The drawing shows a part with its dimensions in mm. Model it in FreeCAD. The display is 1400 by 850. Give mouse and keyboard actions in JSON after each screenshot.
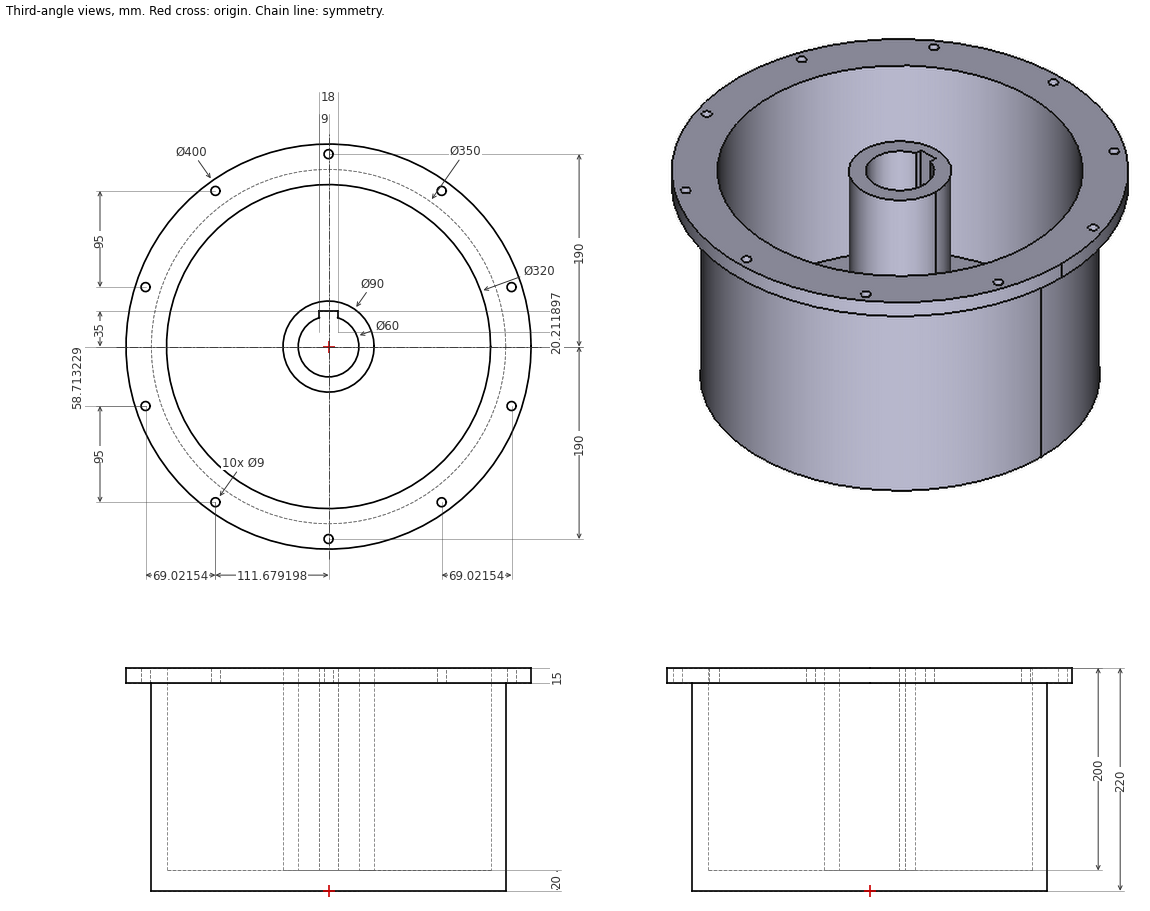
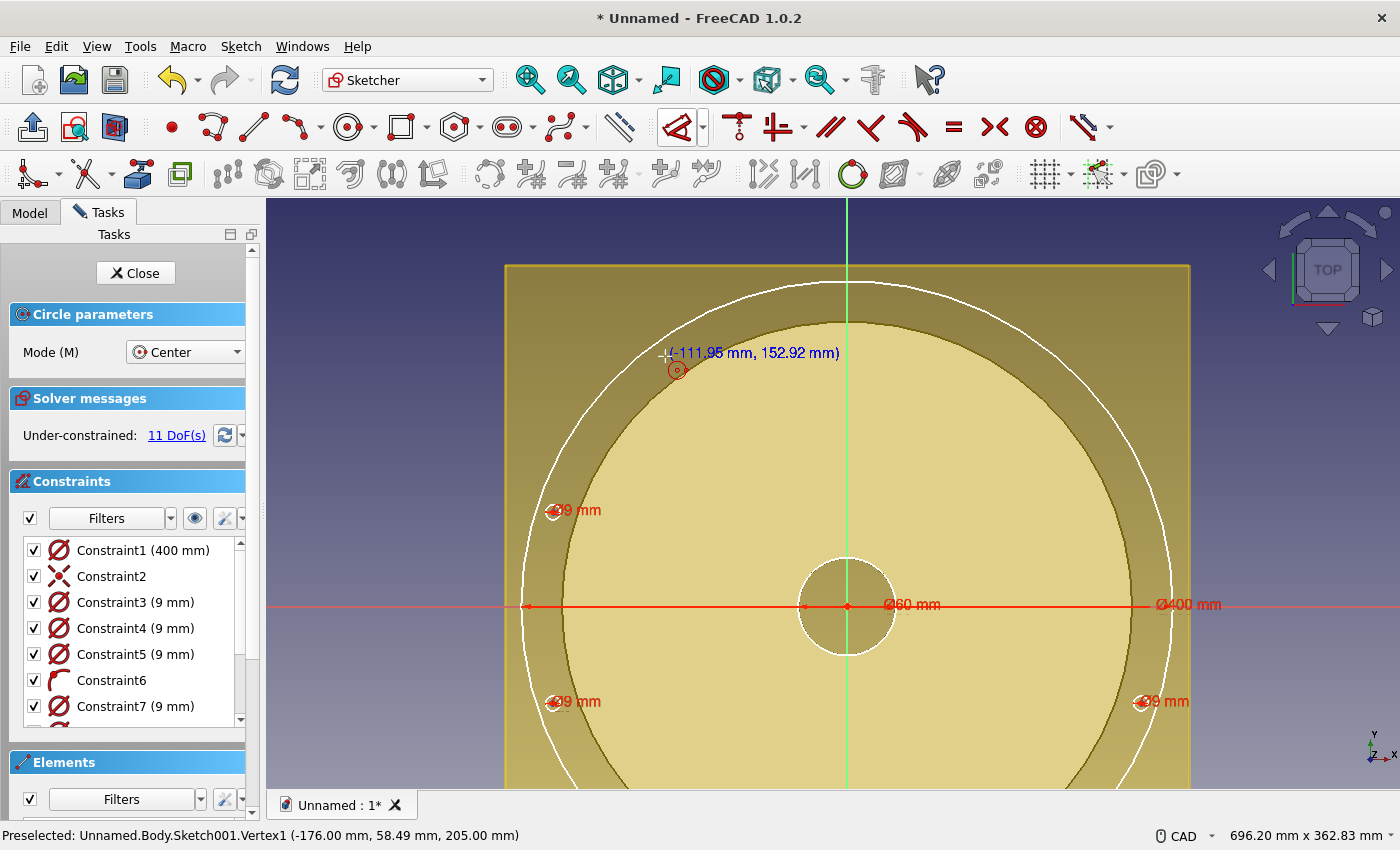
{"action": "left_click", "coordinate": [665, 356]}
{"action": "mouse_move", "coordinate": [670, 351]}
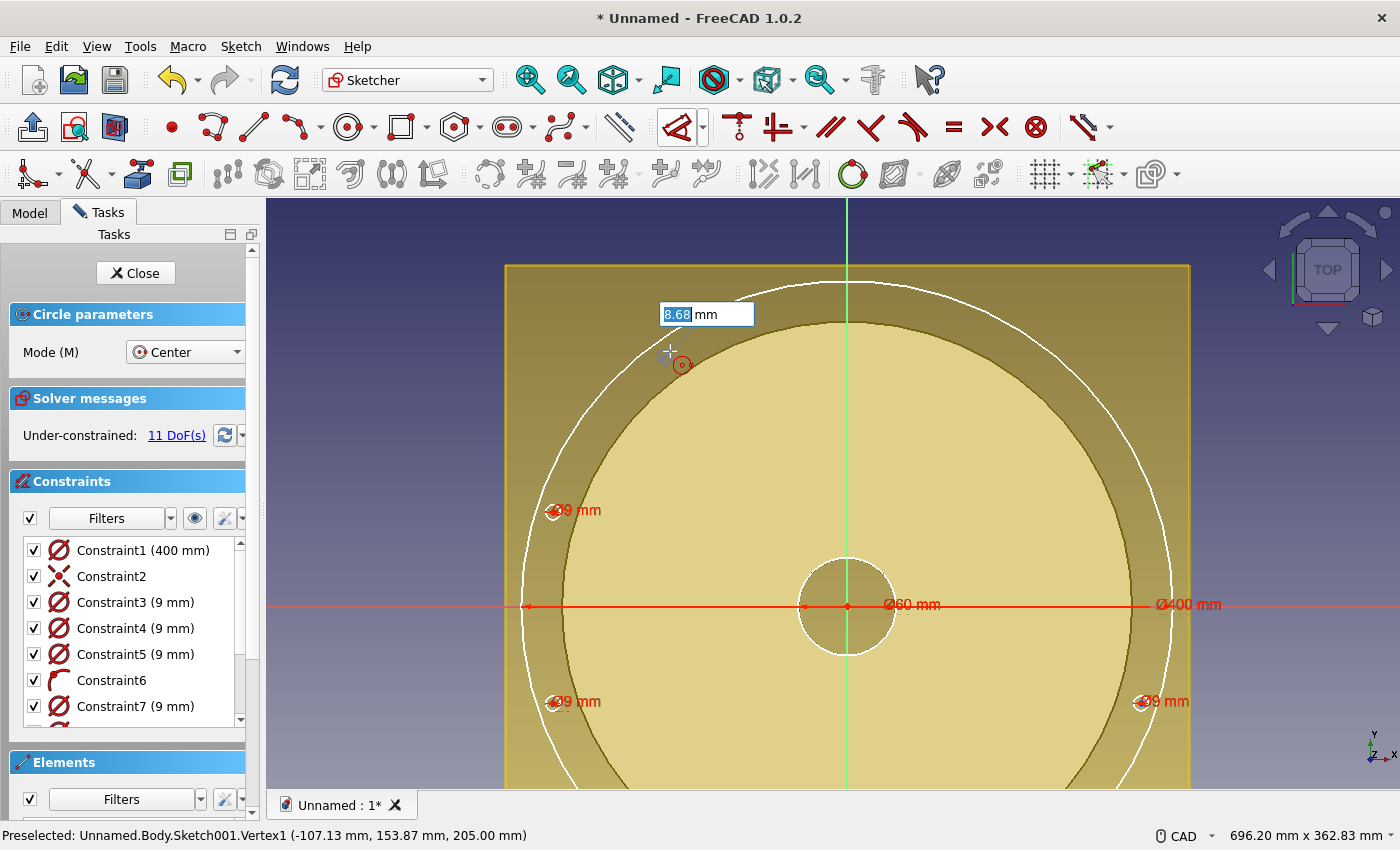
{"action": "type", "text": "9"}
{"action": "key", "text": "Return"}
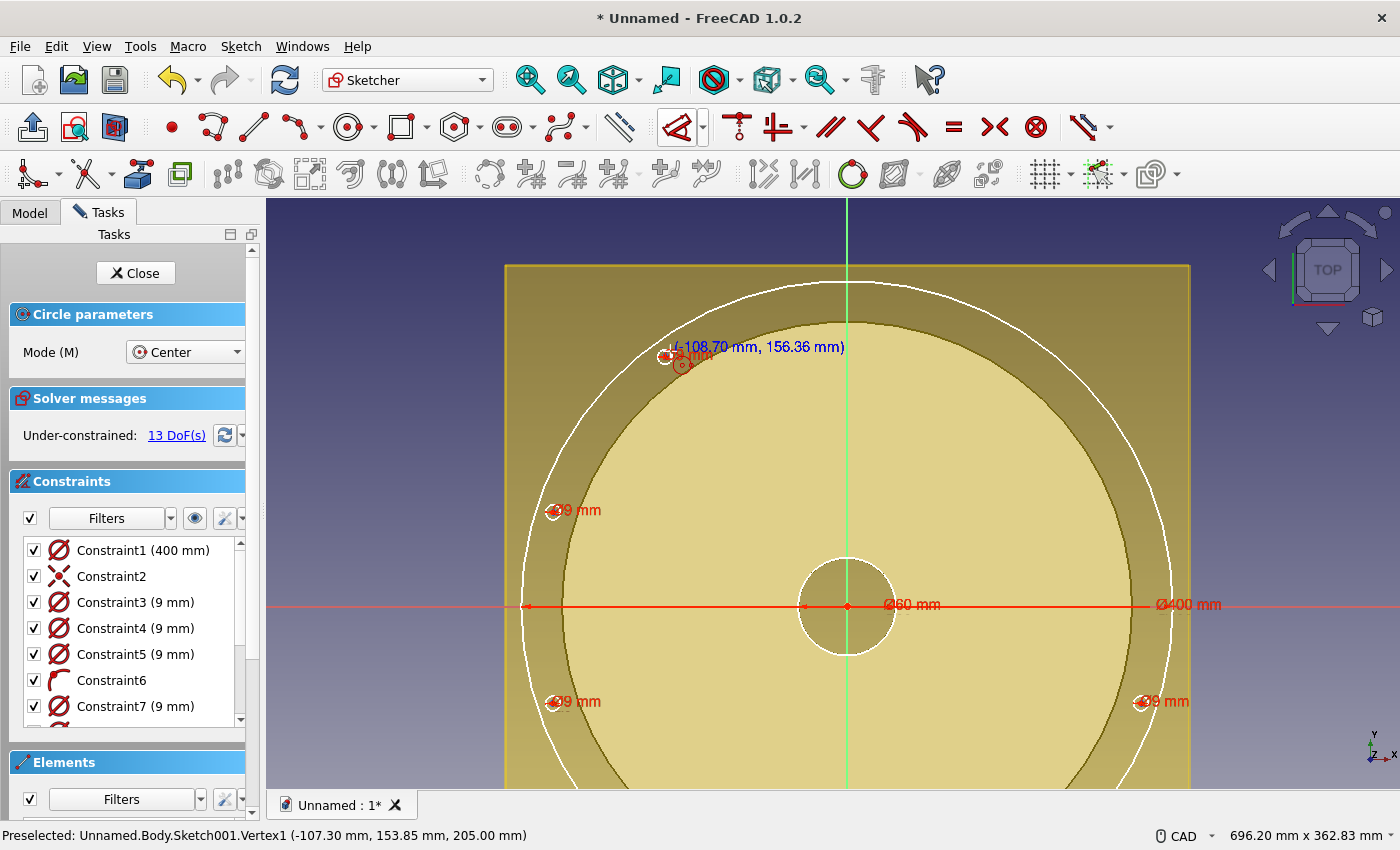
{"action": "scroll", "coordinate": [1141, 511], "scroll_direction": "up", "scroll_amount": 6}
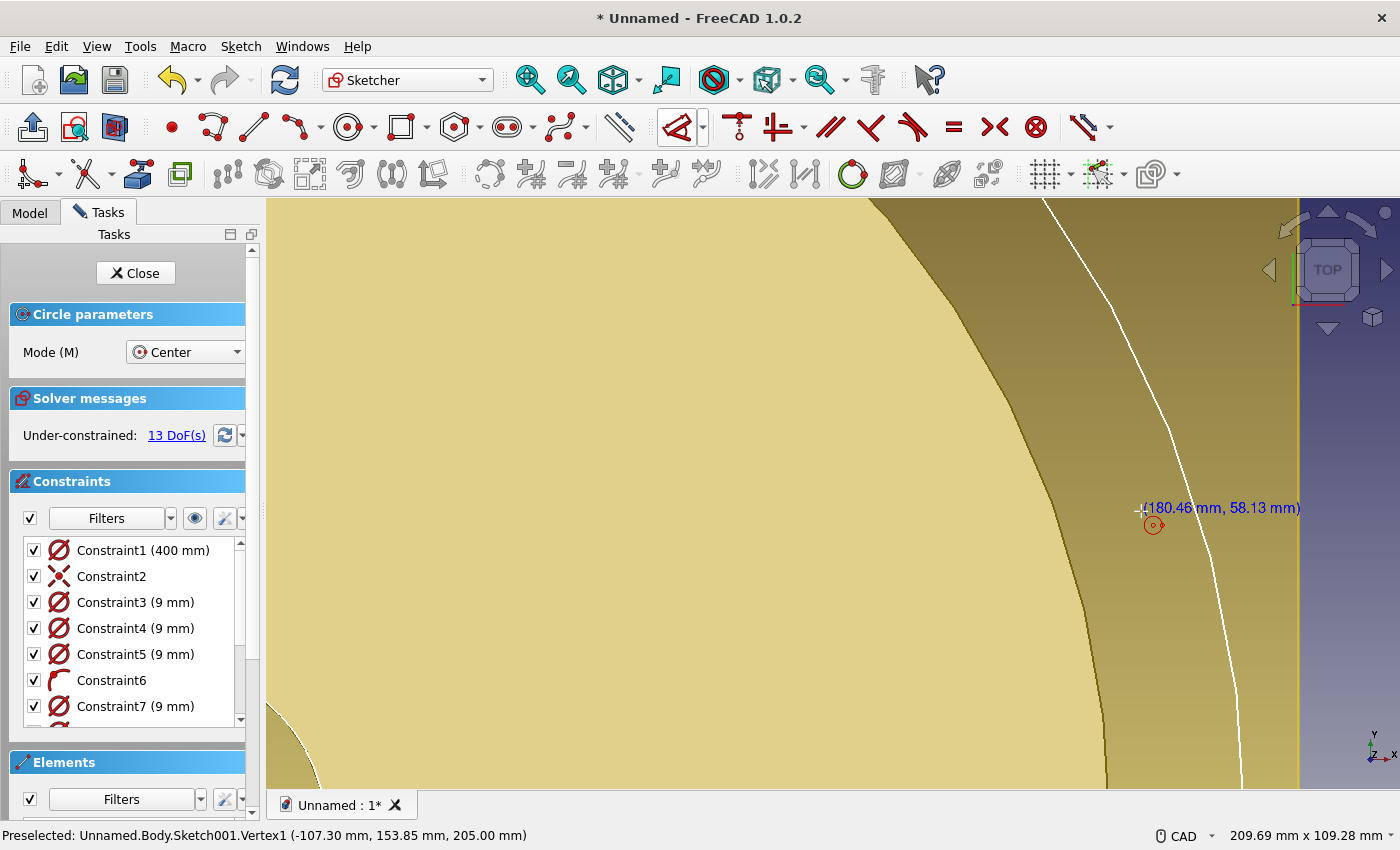
{"action": "scroll", "coordinate": [884, 427], "scroll_direction": "down", "scroll_amount": 9}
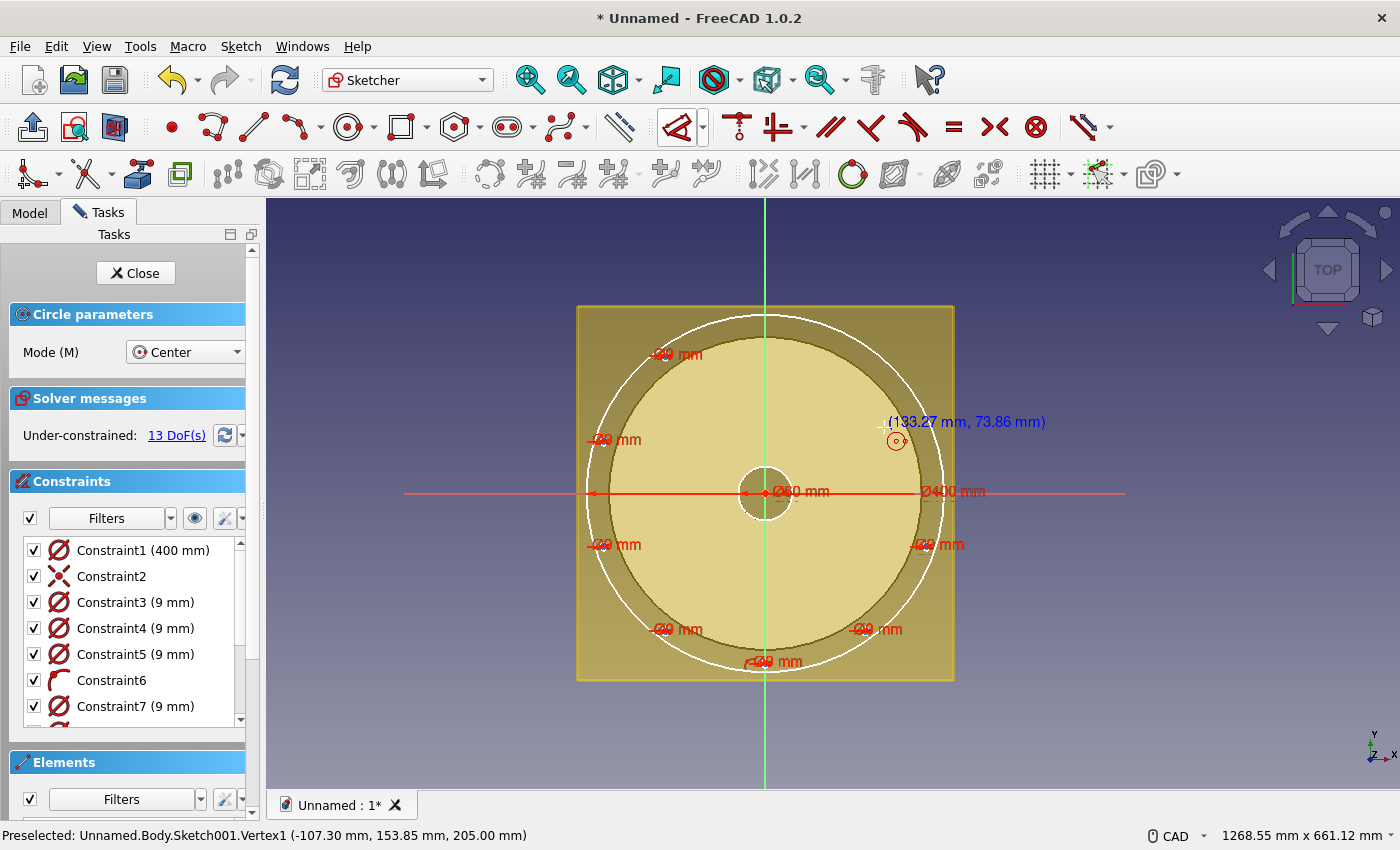
{"action": "scroll", "coordinate": [927, 441], "scroll_direction": "up", "scroll_amount": 3}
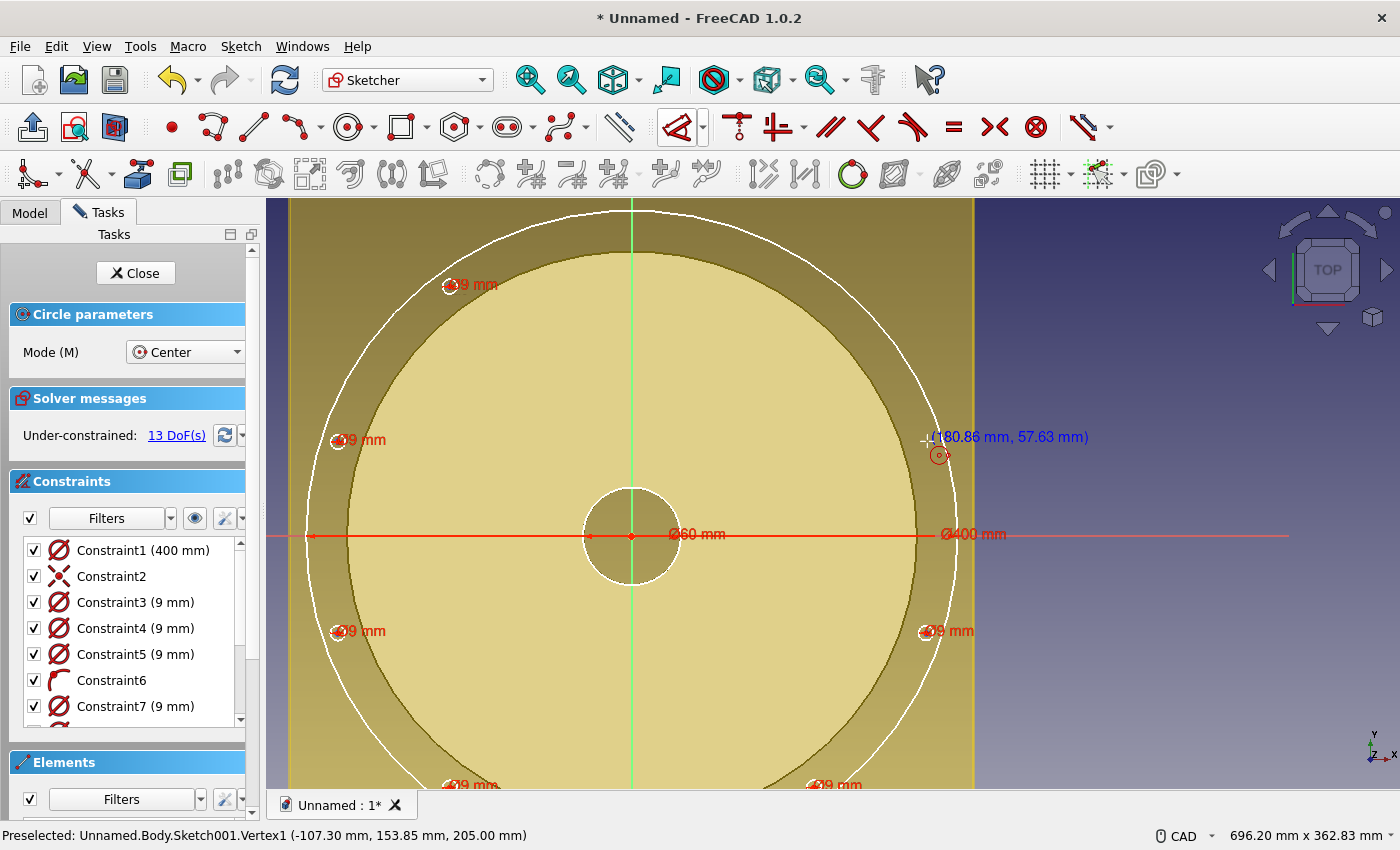
{"action": "left_click", "coordinate": [926, 441]}
{"action": "mouse_move", "coordinate": [921, 436]}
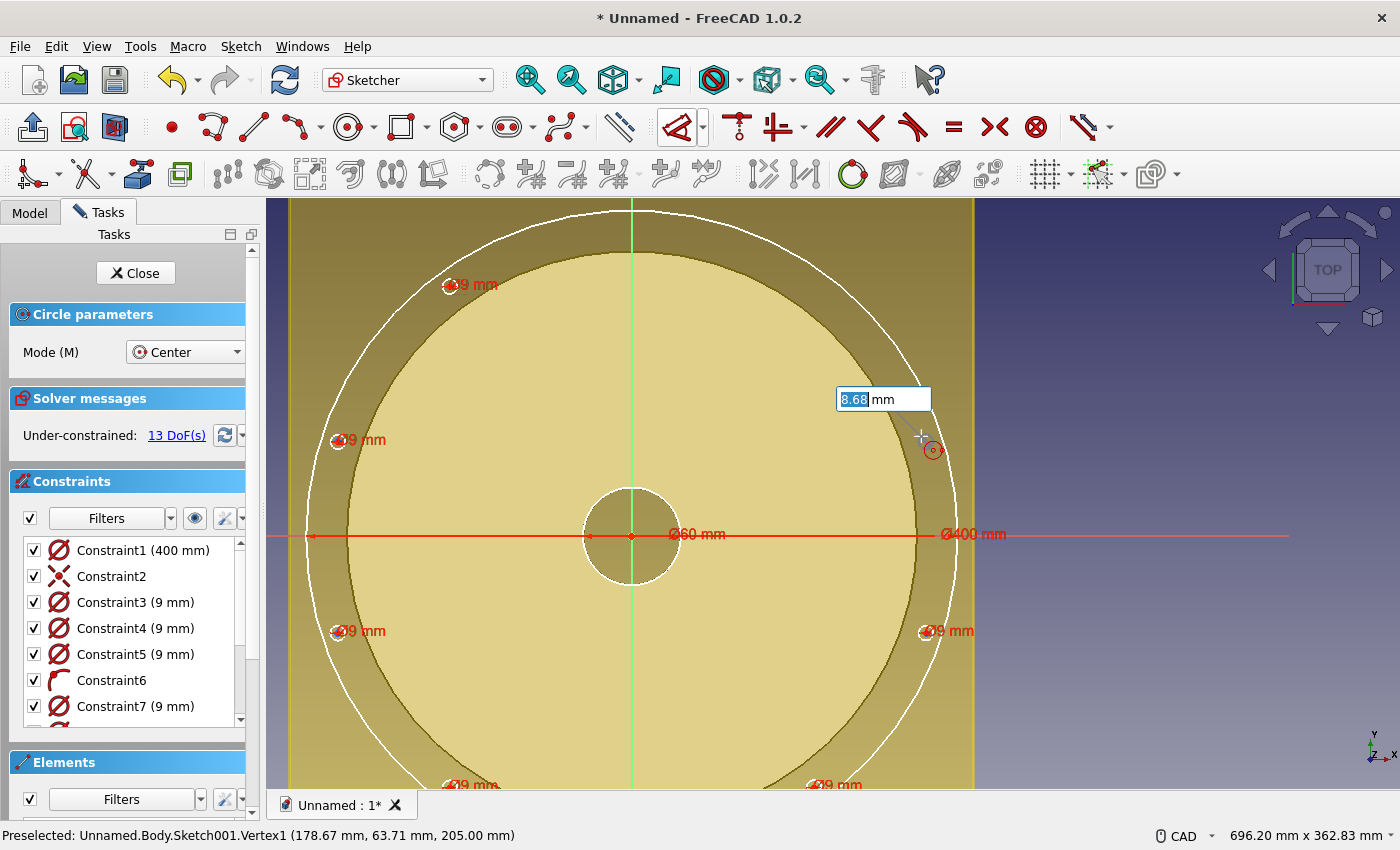
{"action": "type", "text": "9"}
{"action": "key", "text": "Return"}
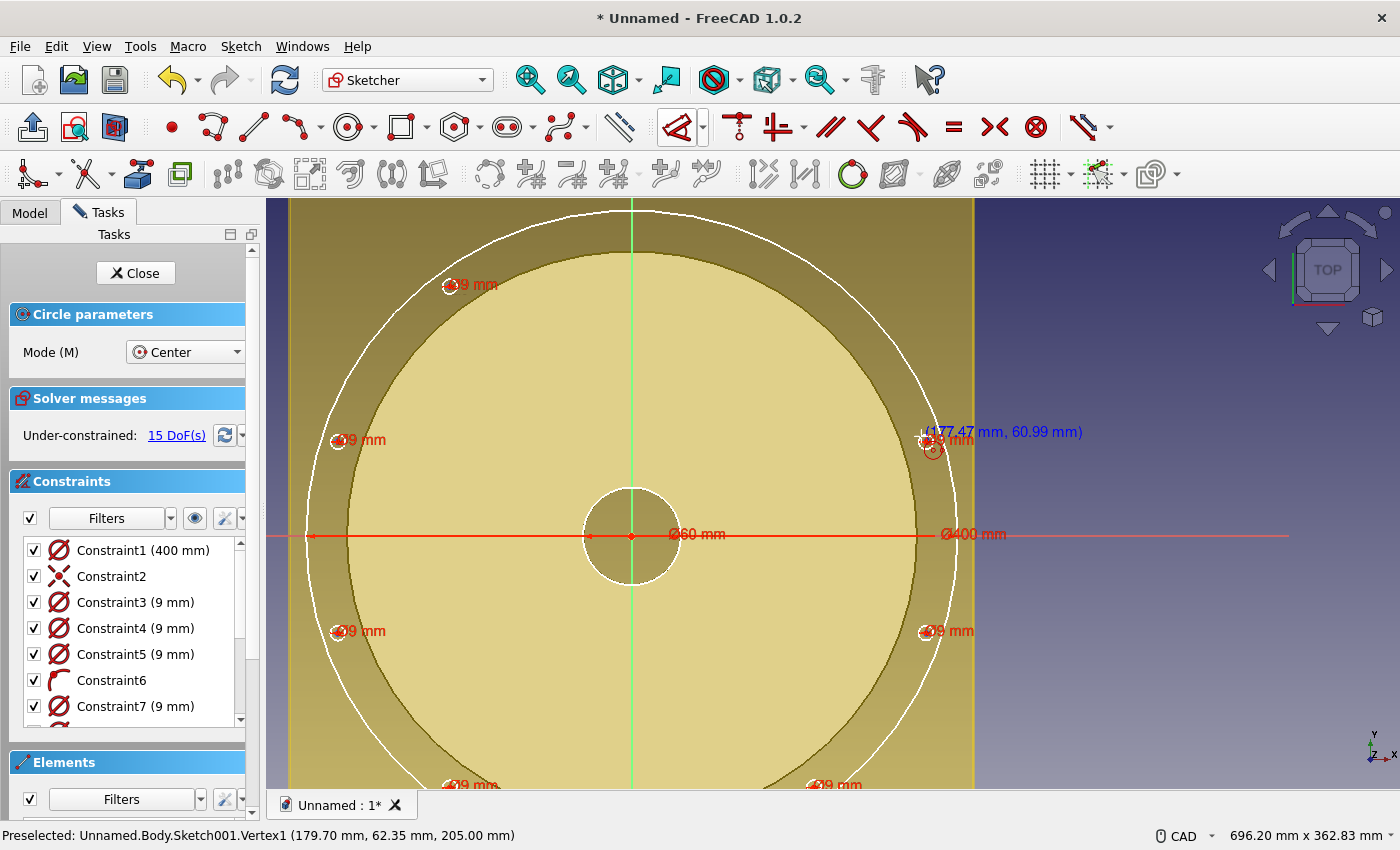
{"action": "scroll", "coordinate": [632, 227], "scroll_direction": "up", "scroll_amount": 6}